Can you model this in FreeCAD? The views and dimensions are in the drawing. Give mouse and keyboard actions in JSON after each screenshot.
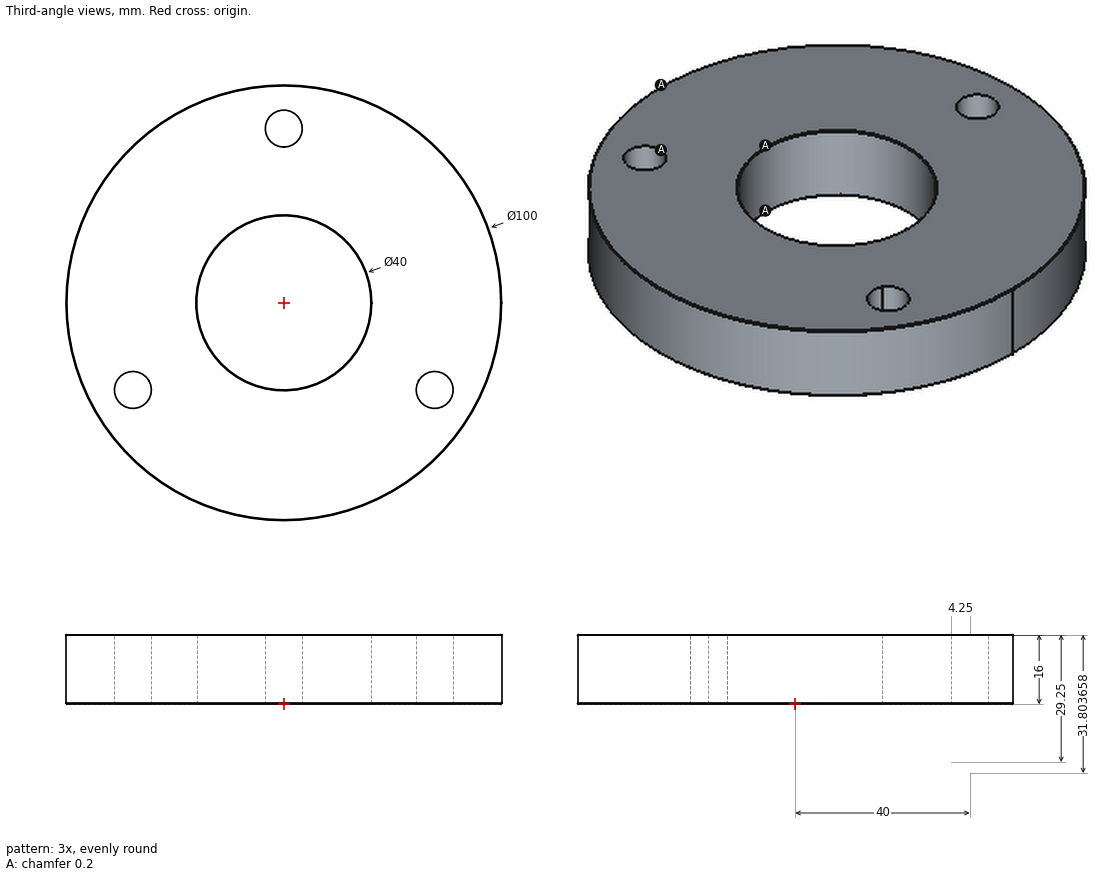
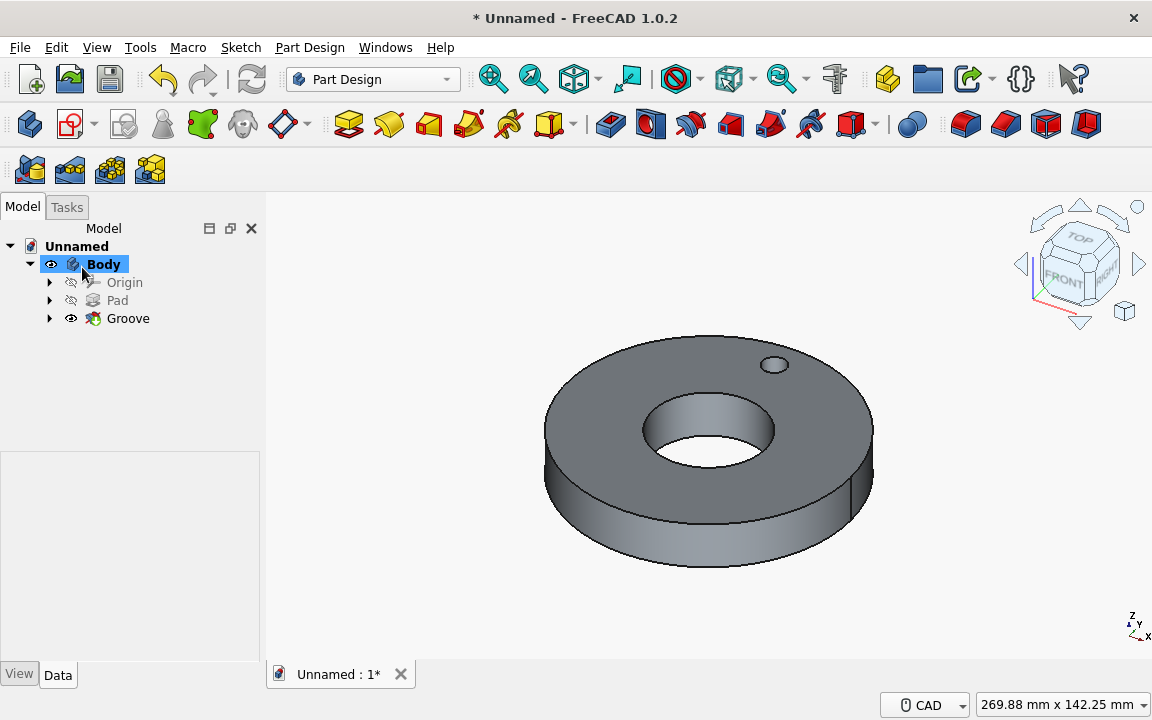
{"action": "left_click", "coordinate": [116, 318]}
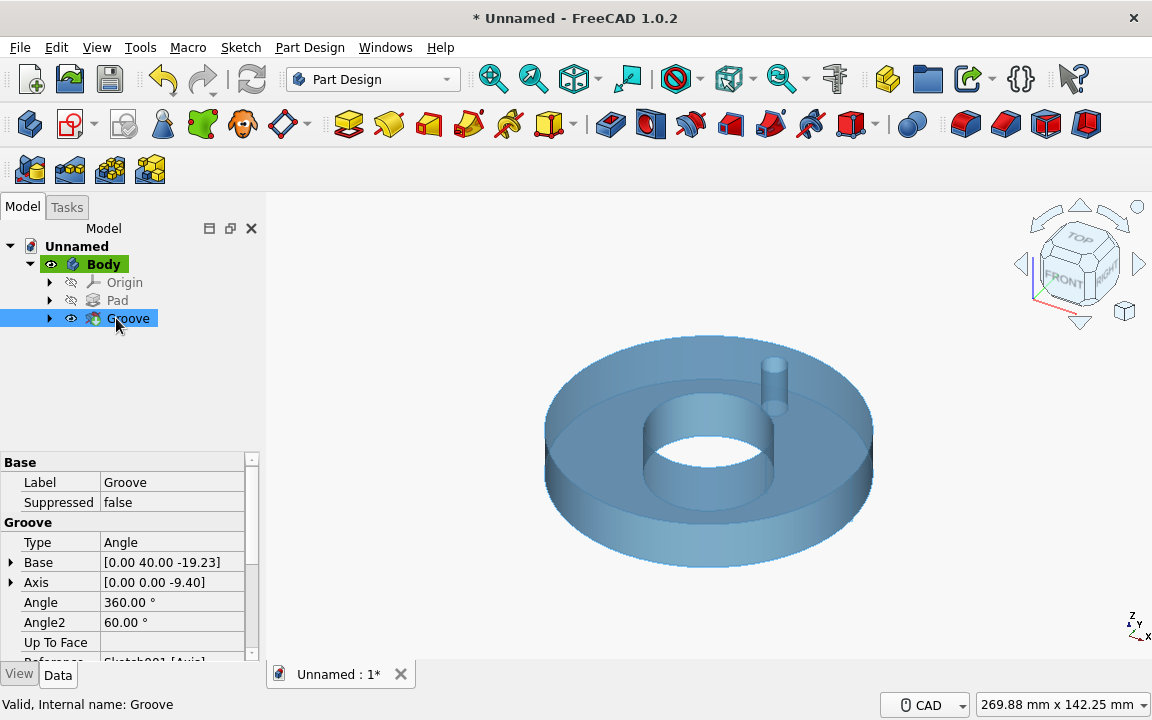
{"action": "left_click", "coordinate": [110, 170]}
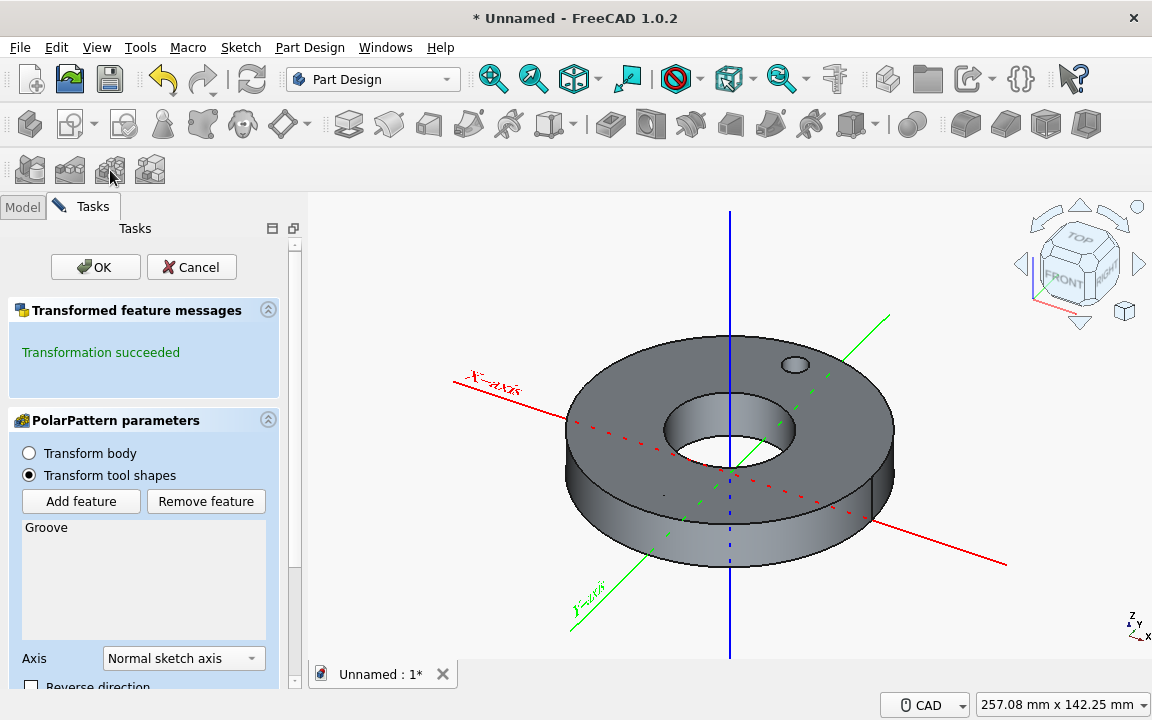
{"action": "left_click", "coordinate": [184, 658]}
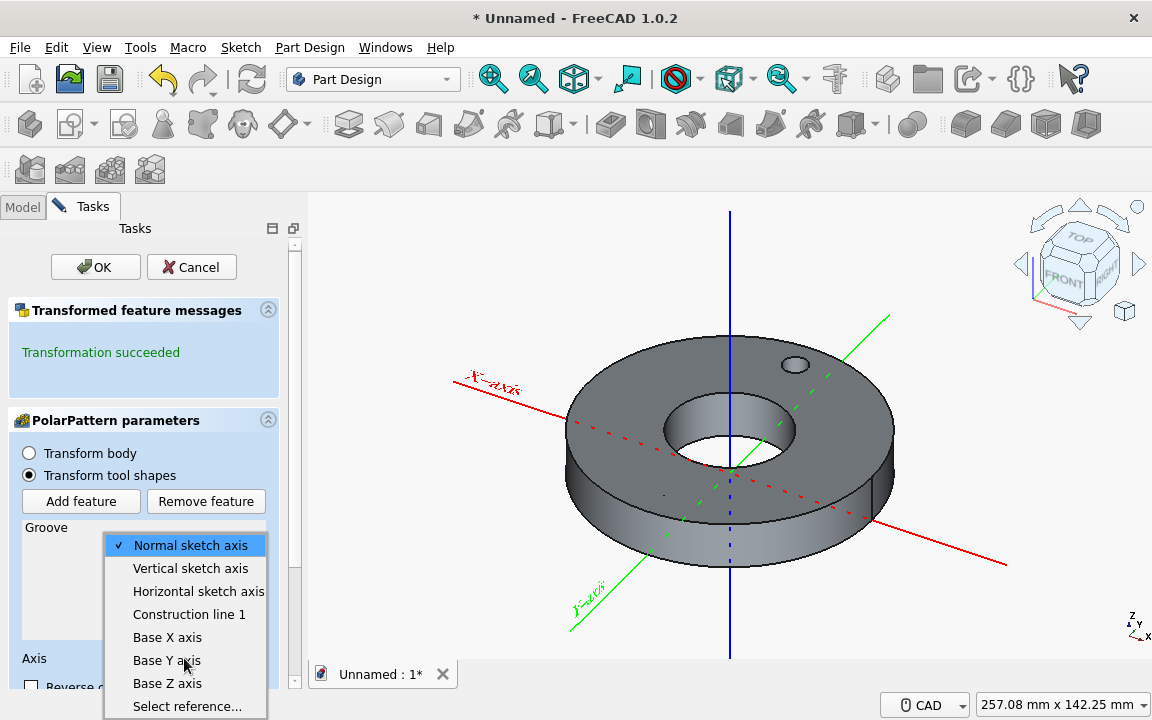
{"action": "left_click", "coordinate": [184, 684]}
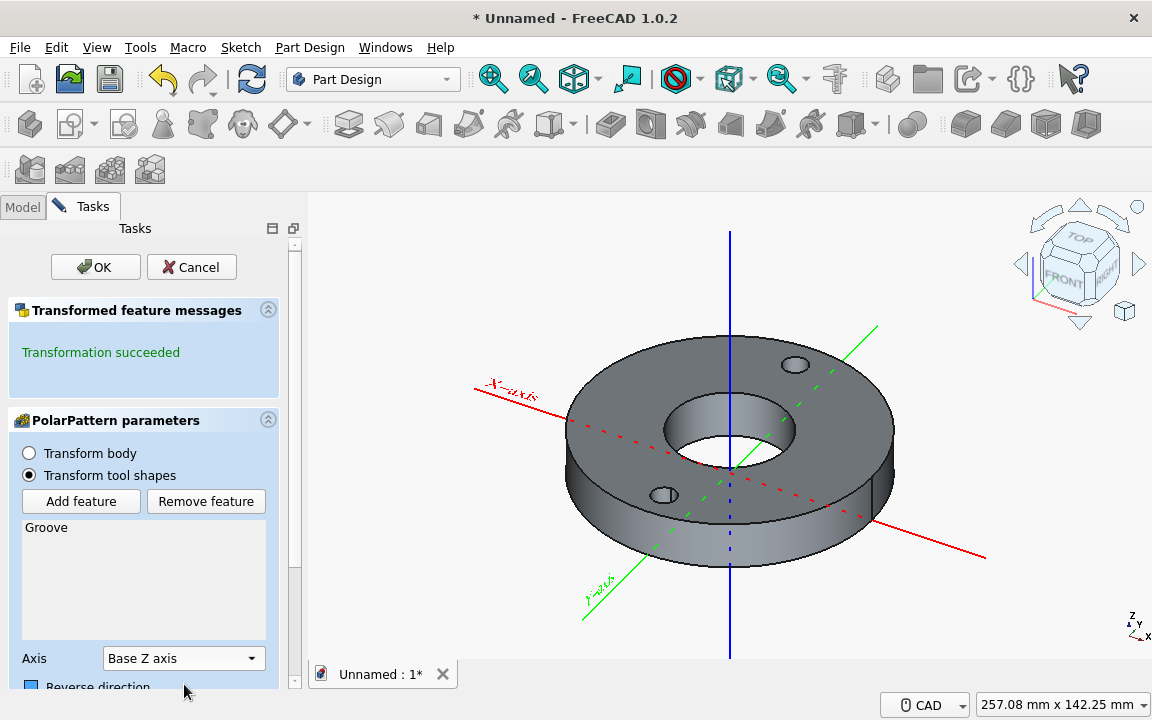
{"action": "scroll", "coordinate": [295, 463], "scroll_direction": "down", "scroll_amount": 3}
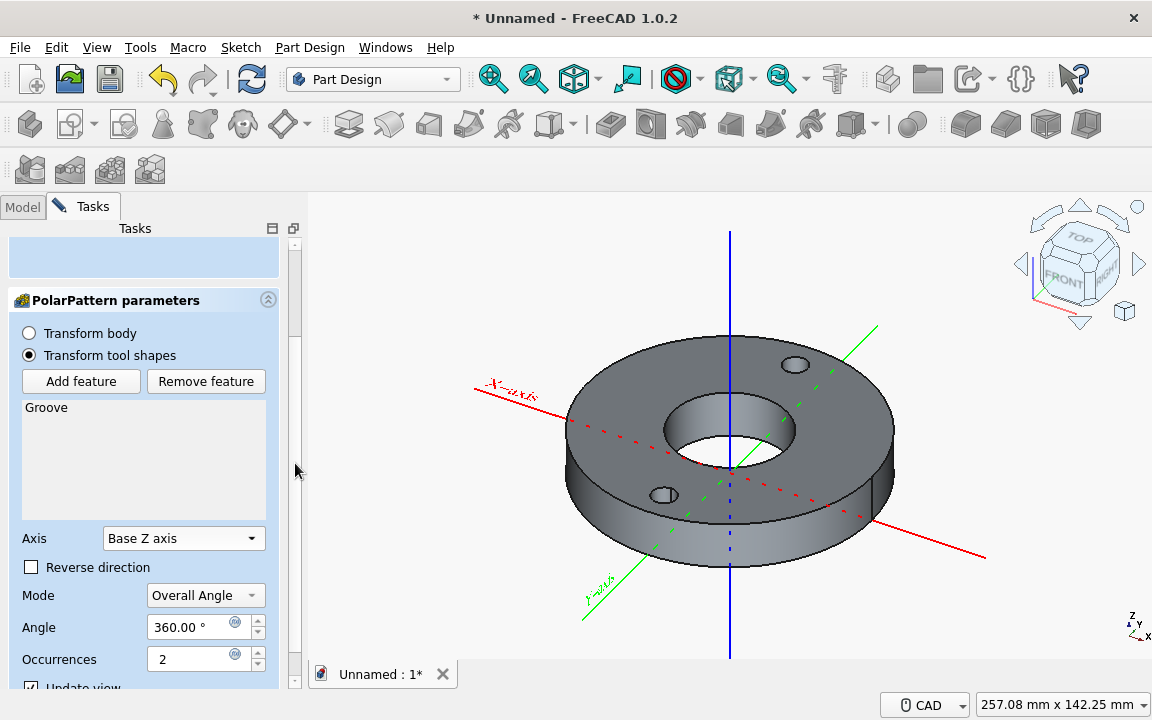
{"action": "triple_click", "coordinate": [198, 628]}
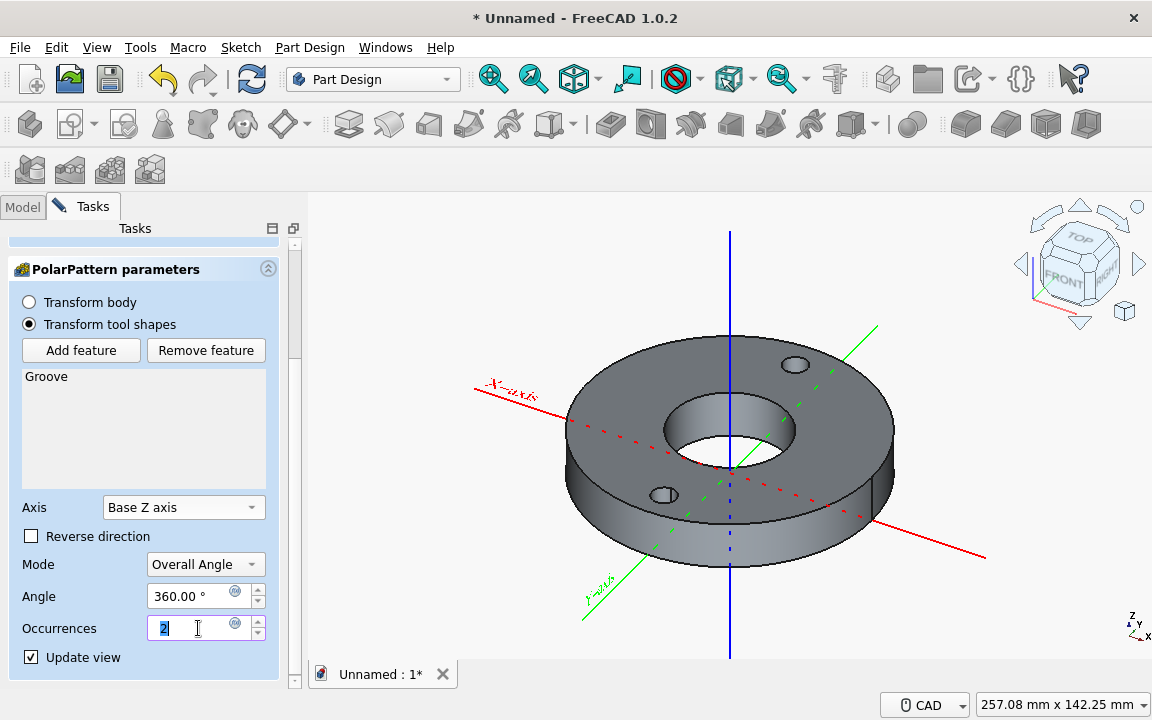
{"action": "type", "text": "3"}
{"action": "key", "text": "Tab"}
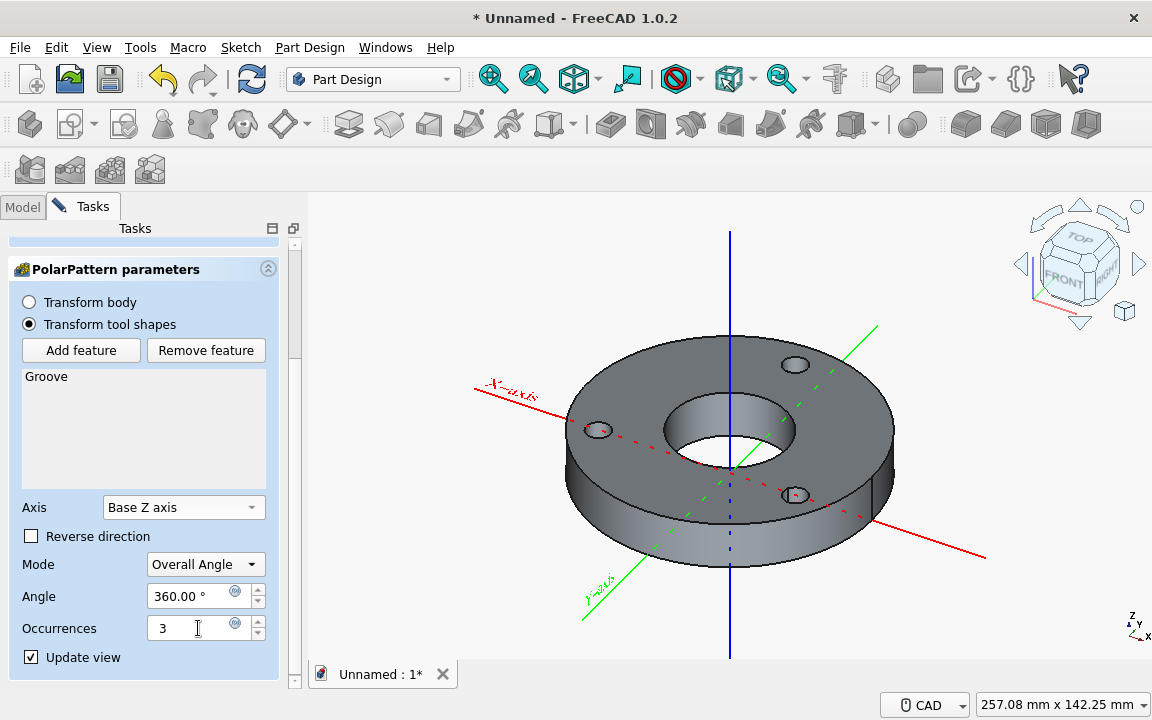
{"action": "scroll", "coordinate": [295, 463], "scroll_direction": "up", "scroll_amount": 4}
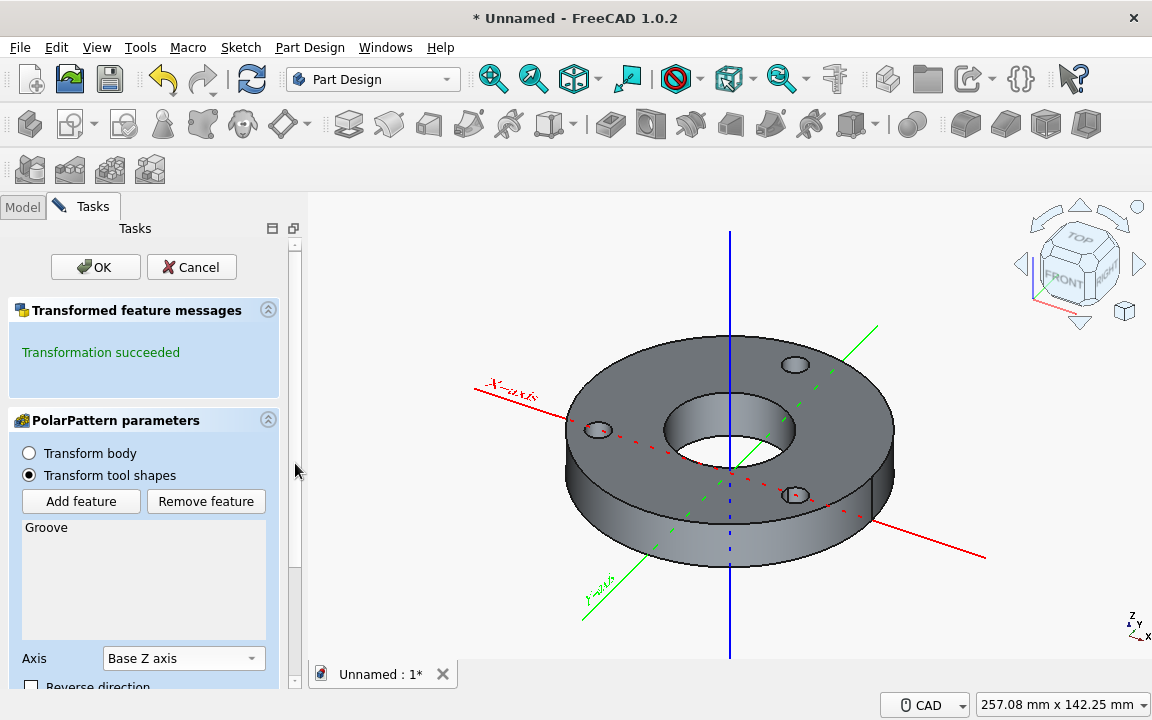
{"action": "left_click", "coordinate": [96, 267]}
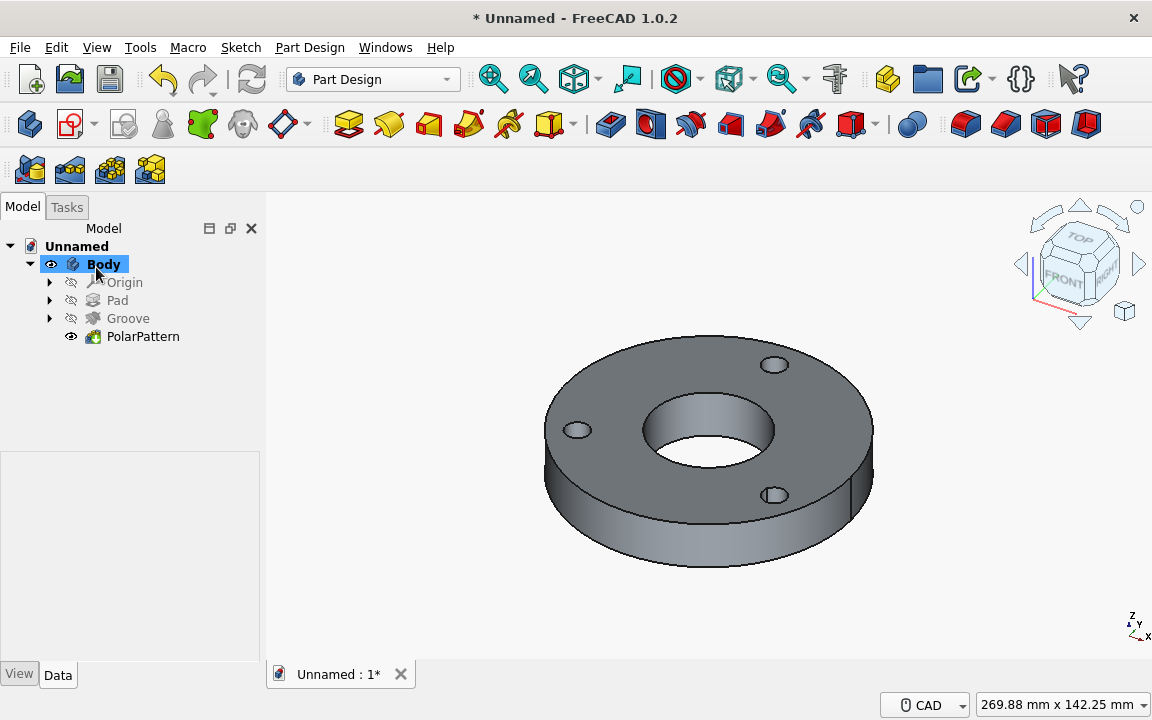
{"action": "left_click", "coordinate": [546, 439]}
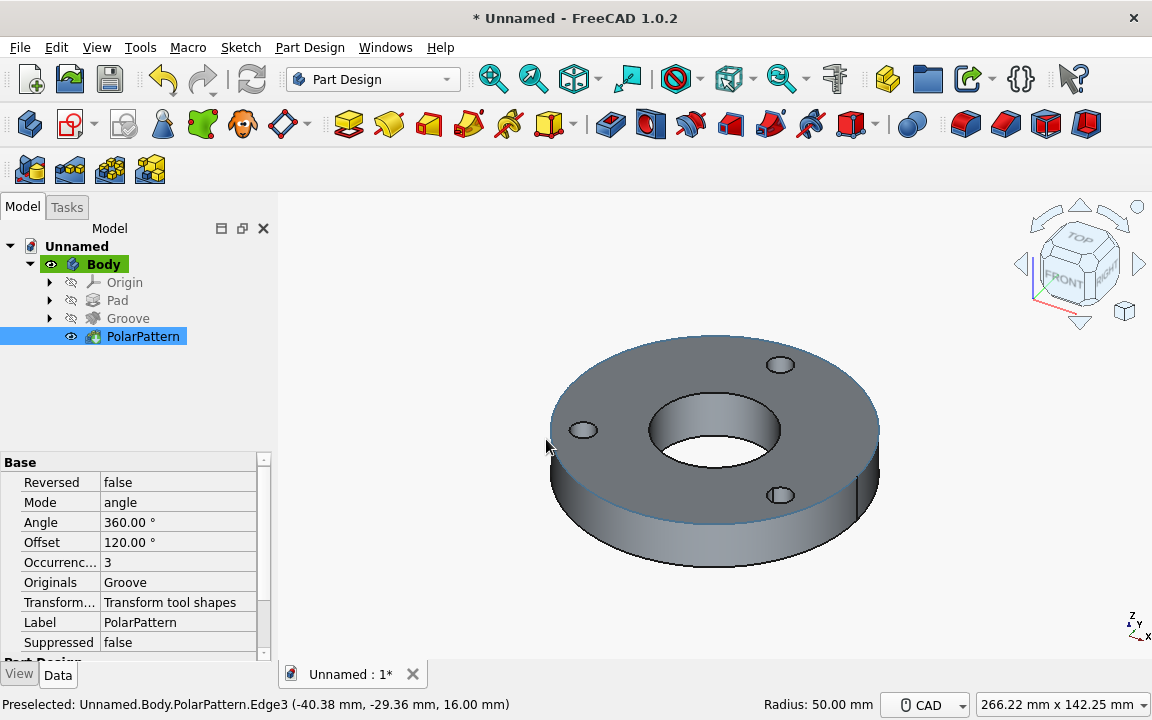
{"action": "left_click", "coordinate": [658, 410], "text": "ctrl"}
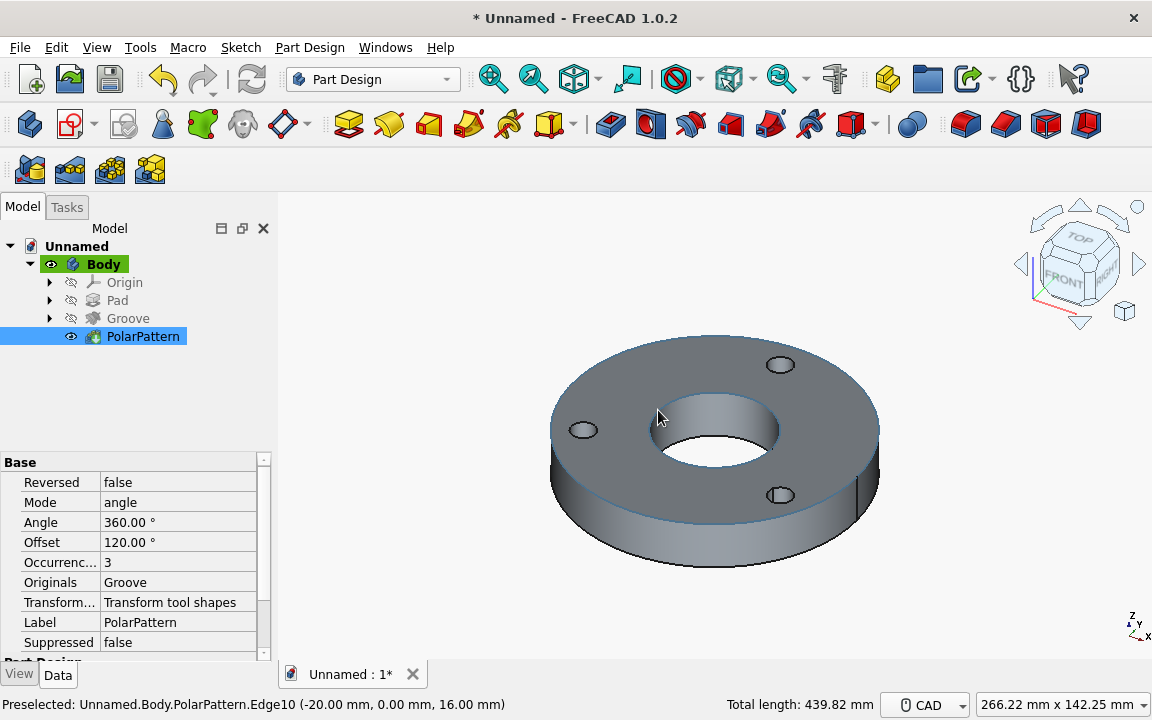
{"action": "key", "text": "0"}